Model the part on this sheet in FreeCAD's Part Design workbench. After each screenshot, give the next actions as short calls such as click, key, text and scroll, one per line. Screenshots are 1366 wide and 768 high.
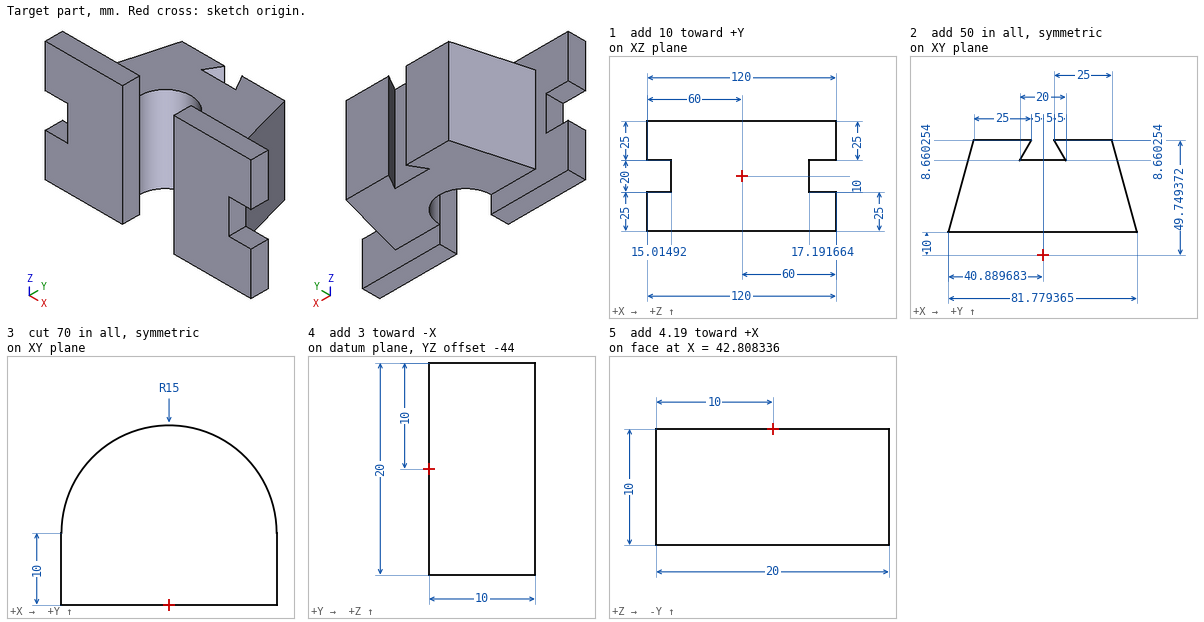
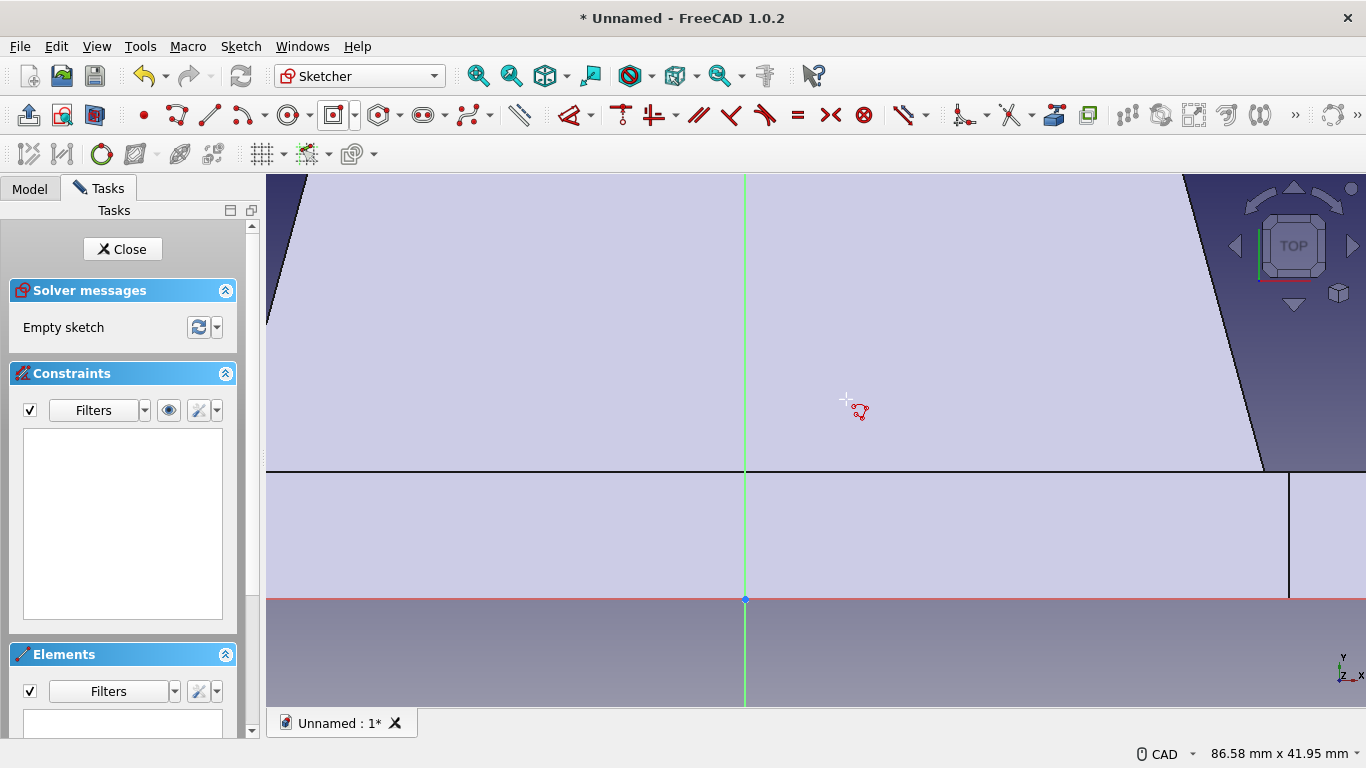
click(555, 472)
click(555, 599)
click(936, 590)
click(936, 472)
right_click(936, 472)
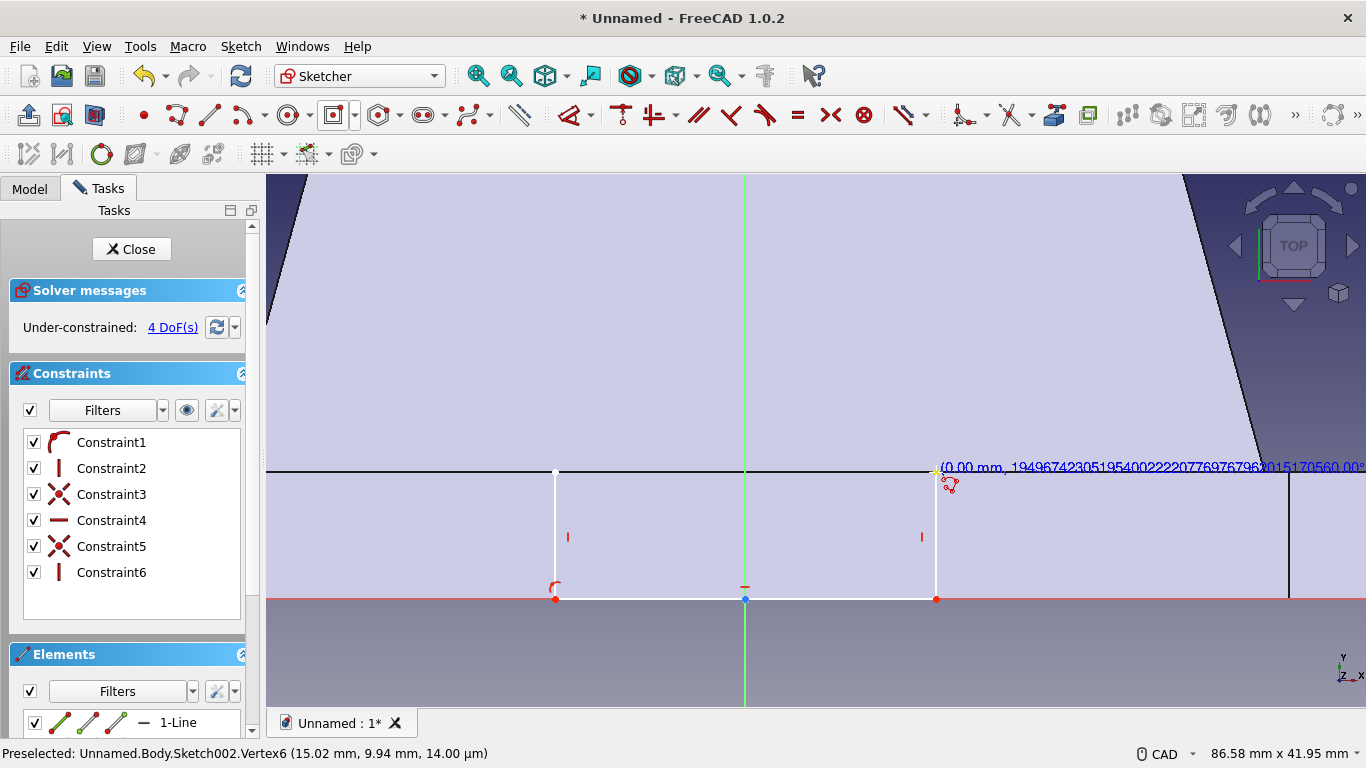
key(g)
key(3)
key(a)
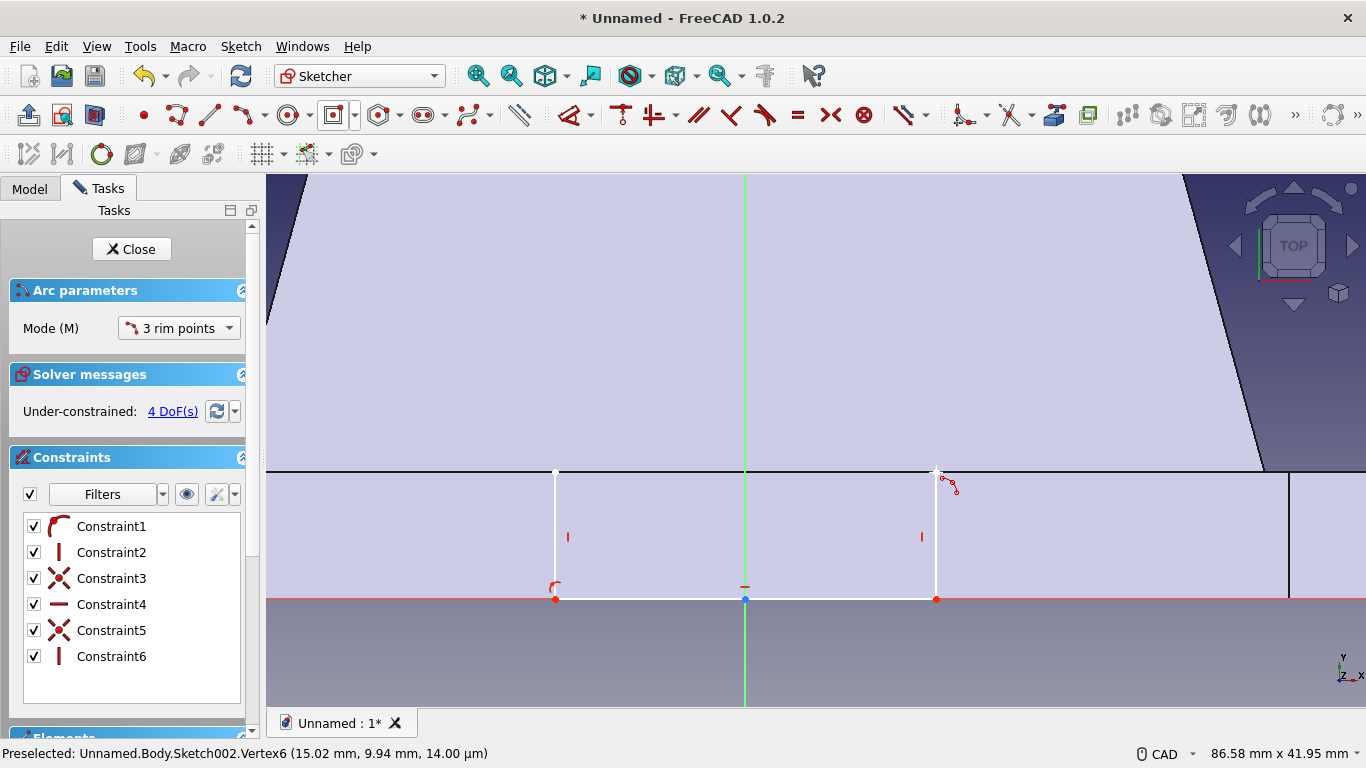
click(936, 473)
click(555, 473)
click(804, 291)
key(Escape)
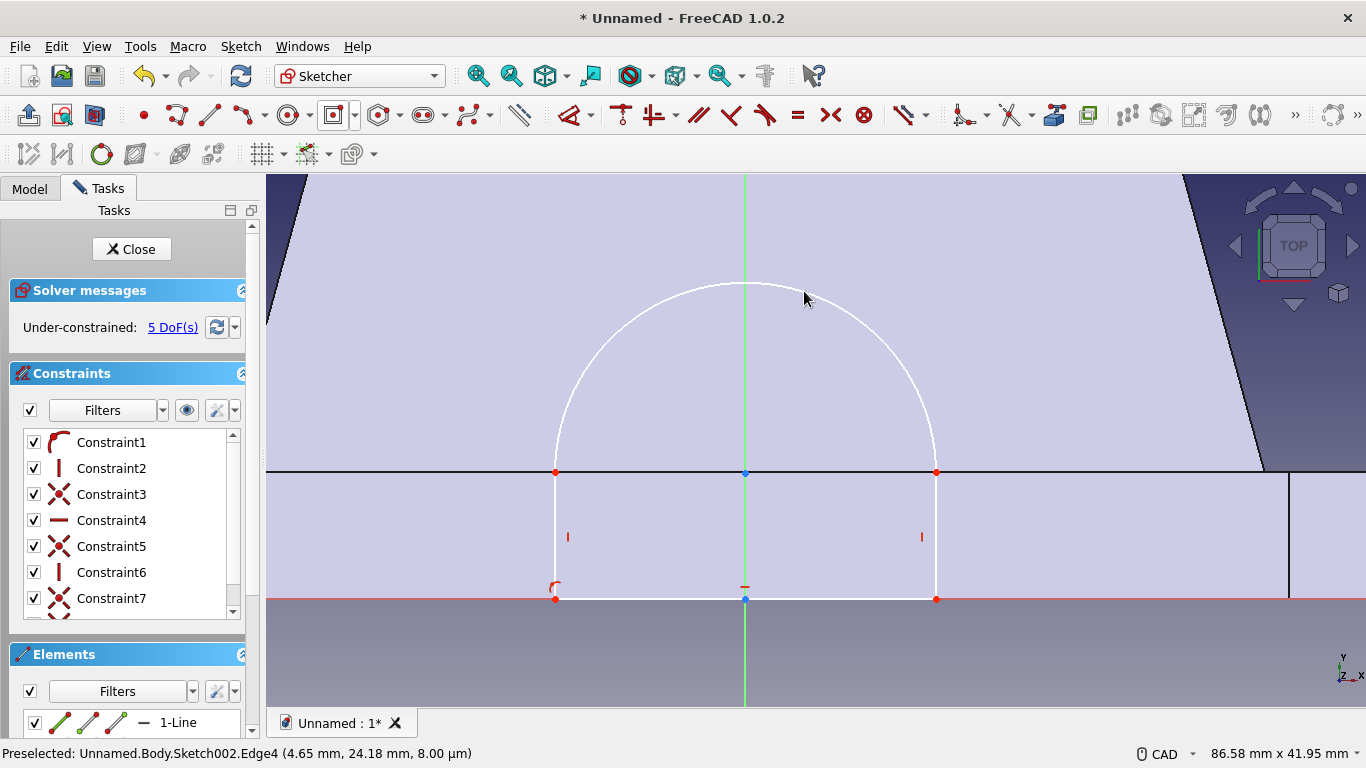
click(555, 511)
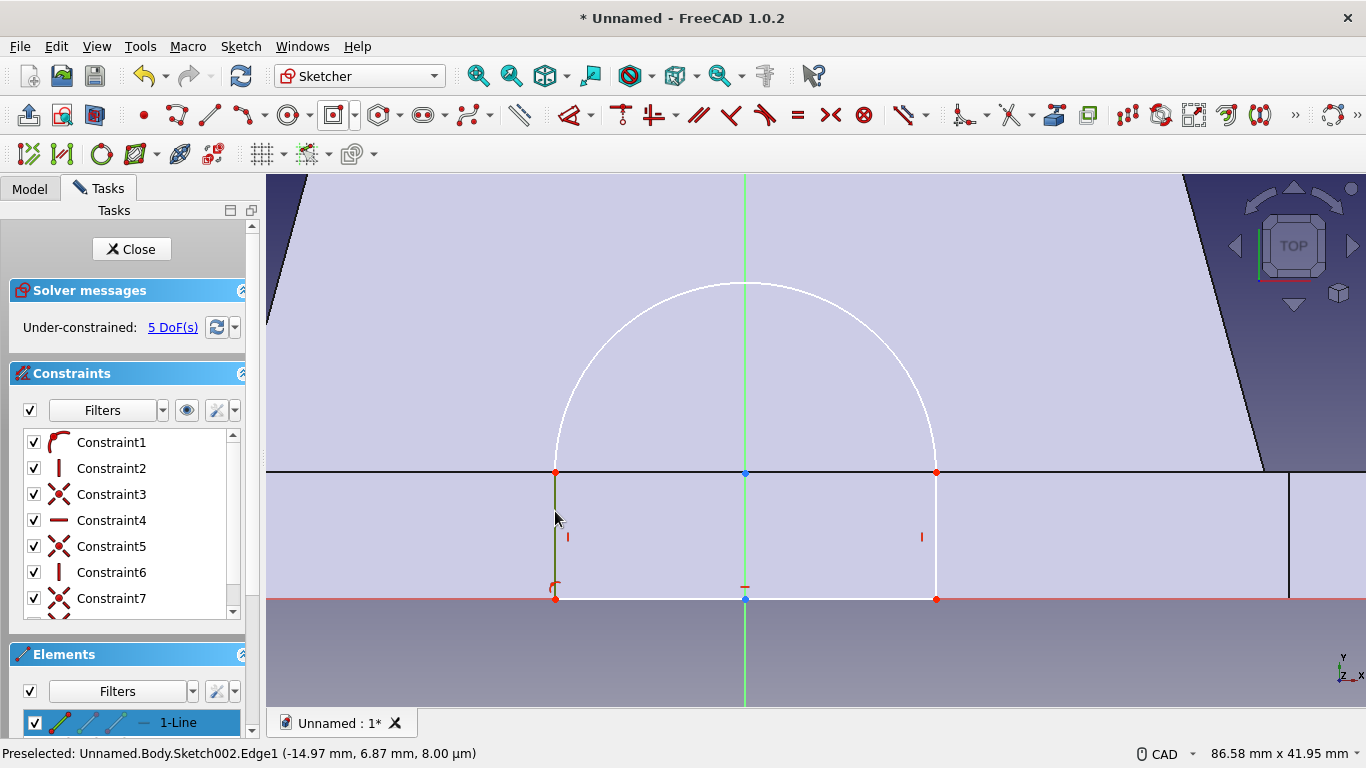
click(857, 319)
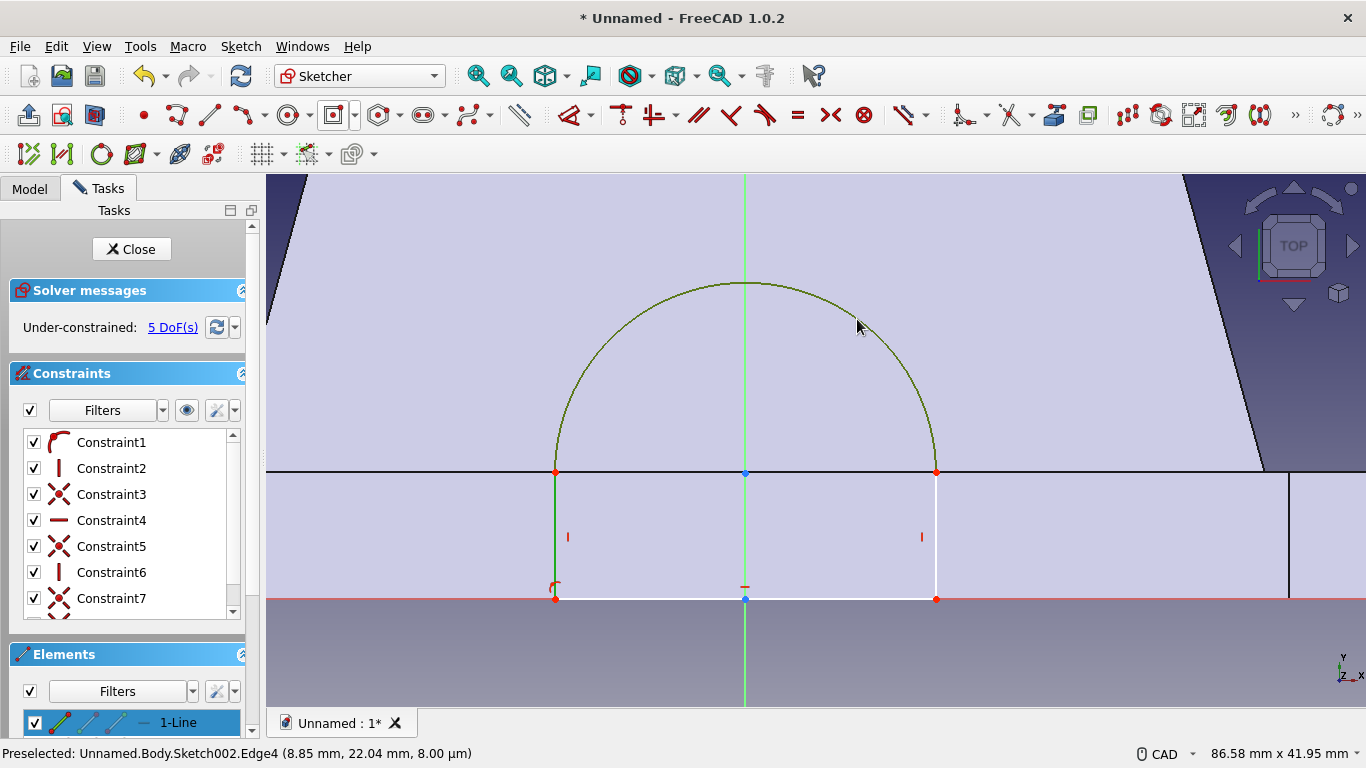
key(t)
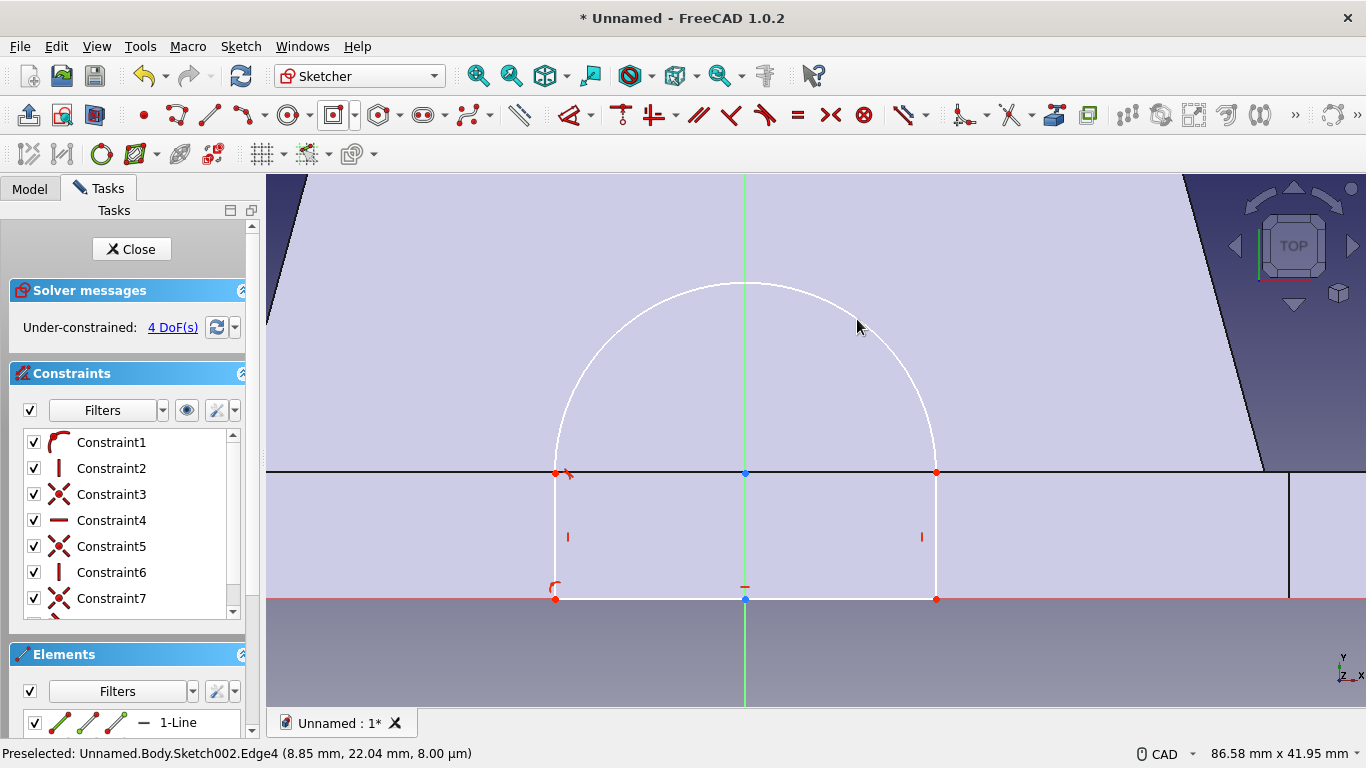
click(936, 561)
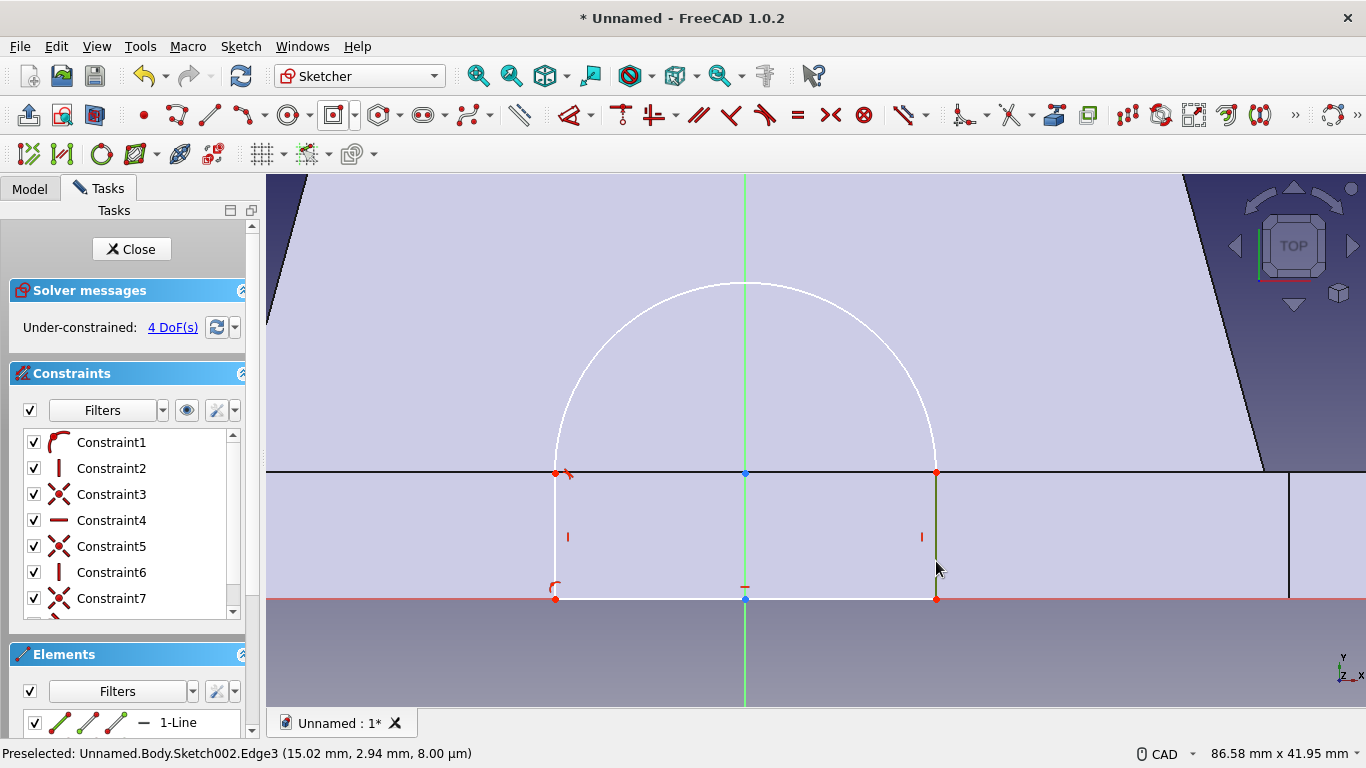
click(857, 319)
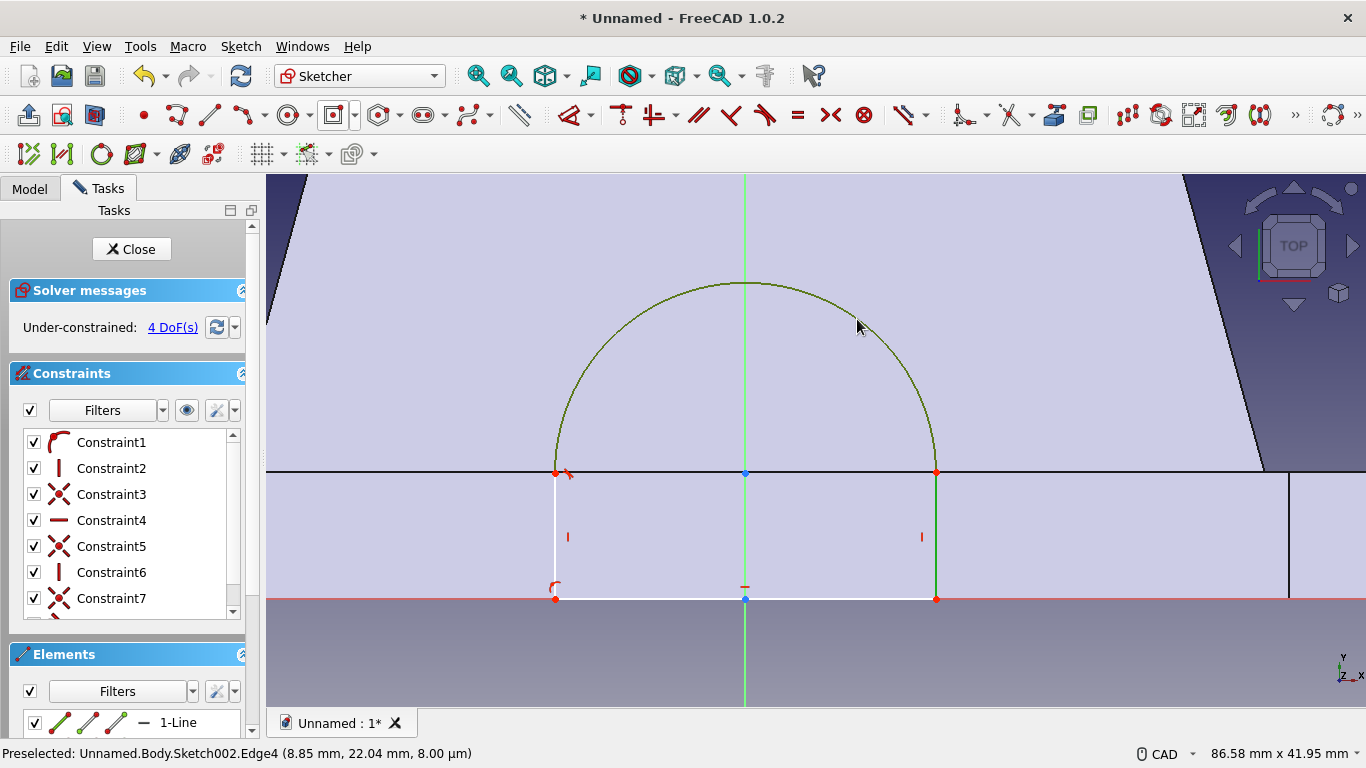
click(765, 116)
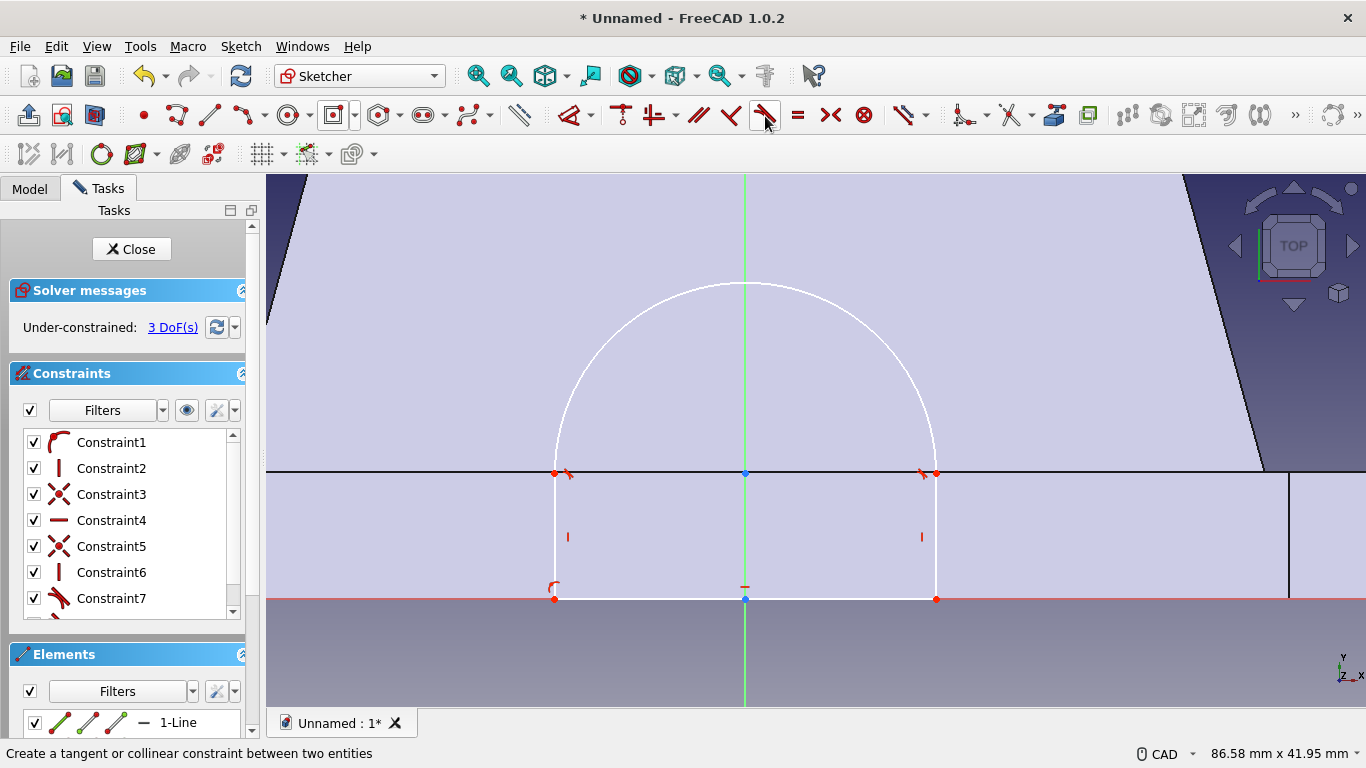
click(745, 473)